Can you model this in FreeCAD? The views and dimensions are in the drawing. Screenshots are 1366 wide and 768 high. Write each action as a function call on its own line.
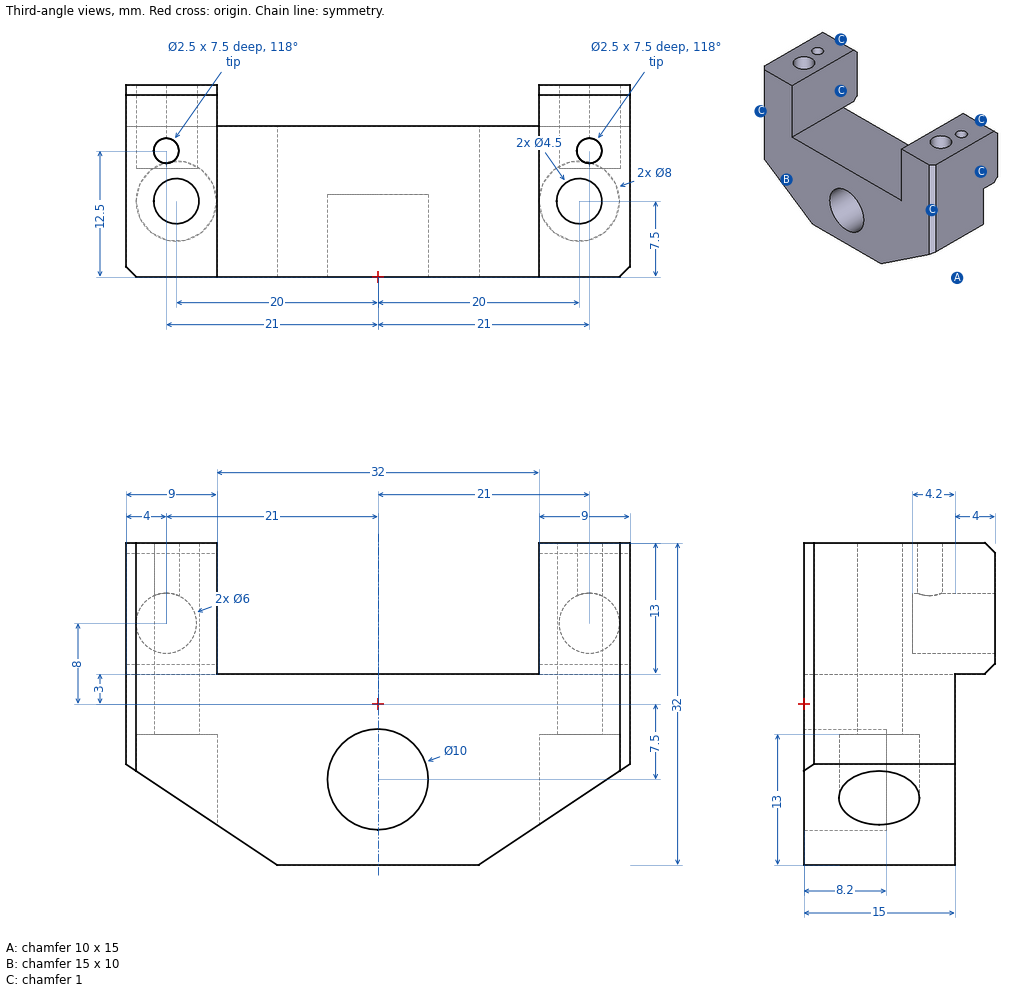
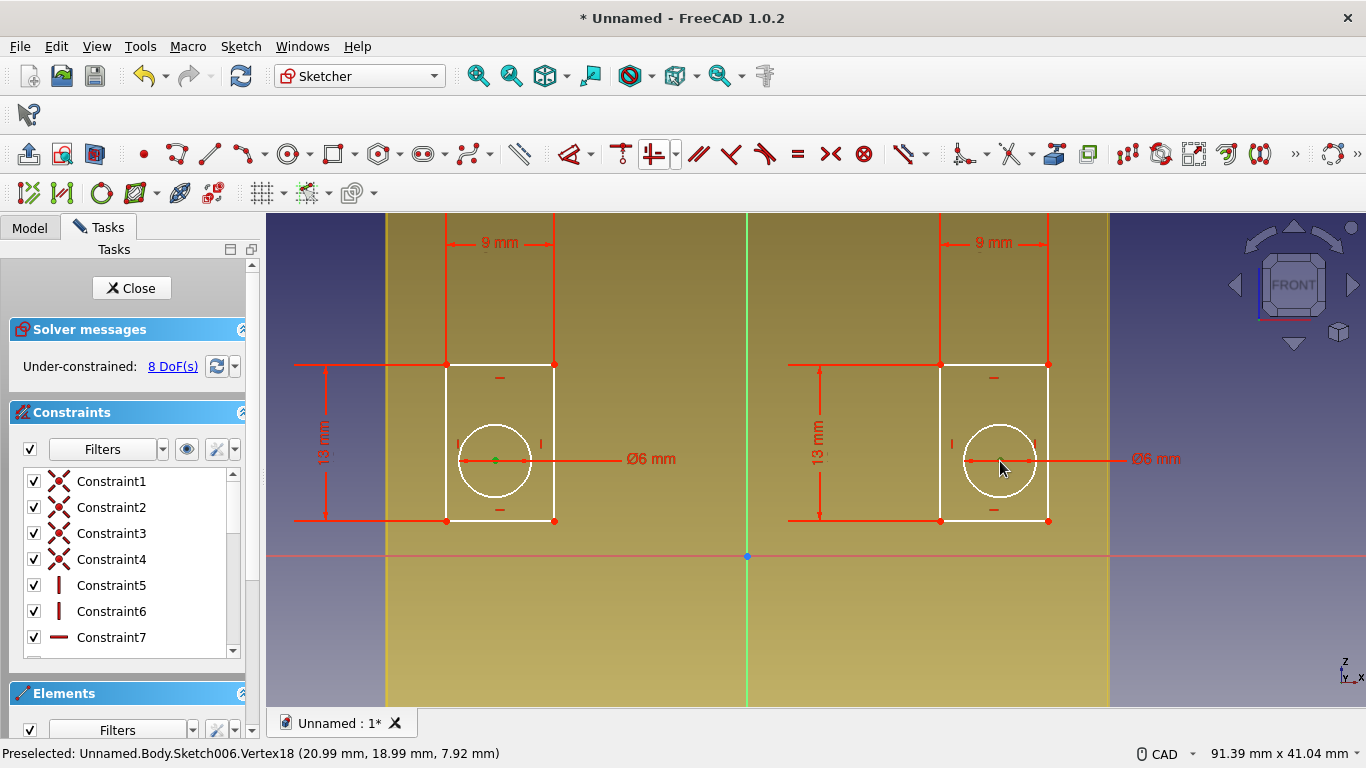
click(747, 648)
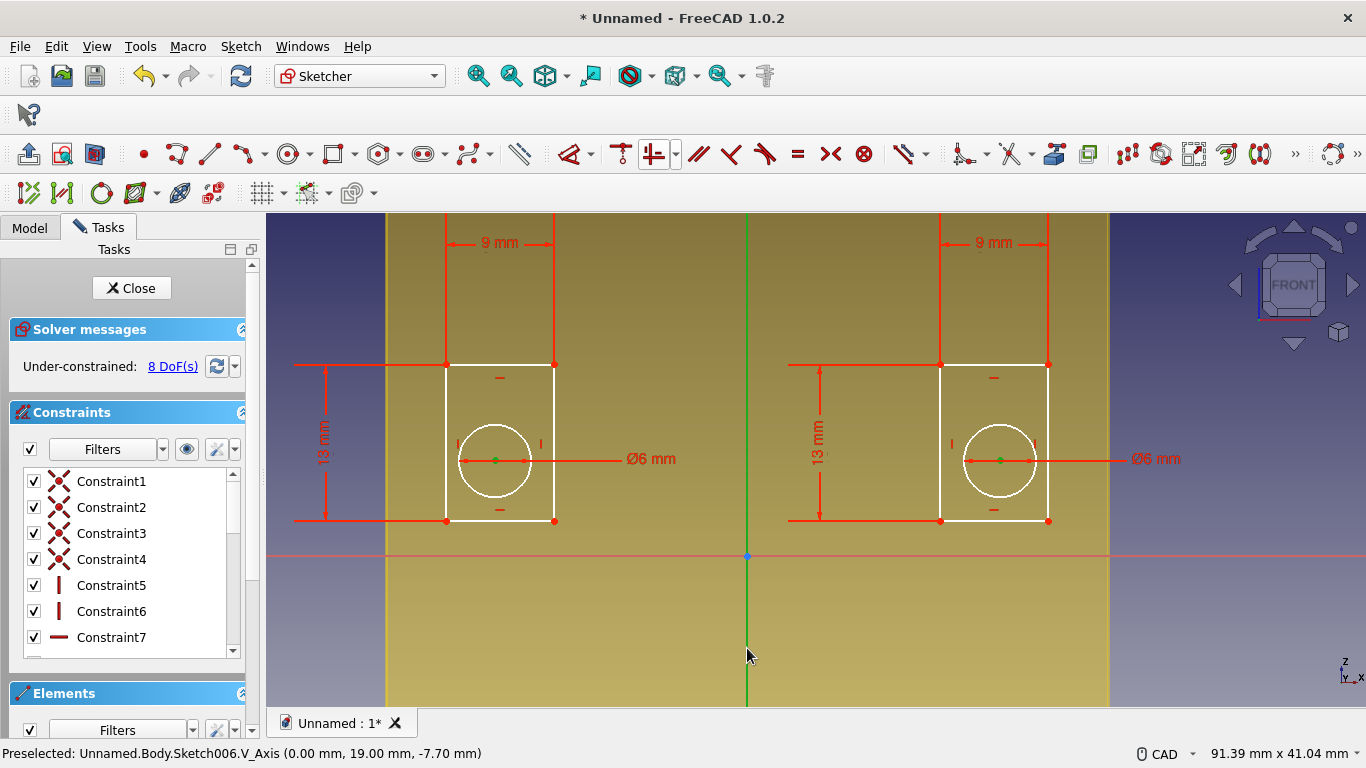
click(831, 154)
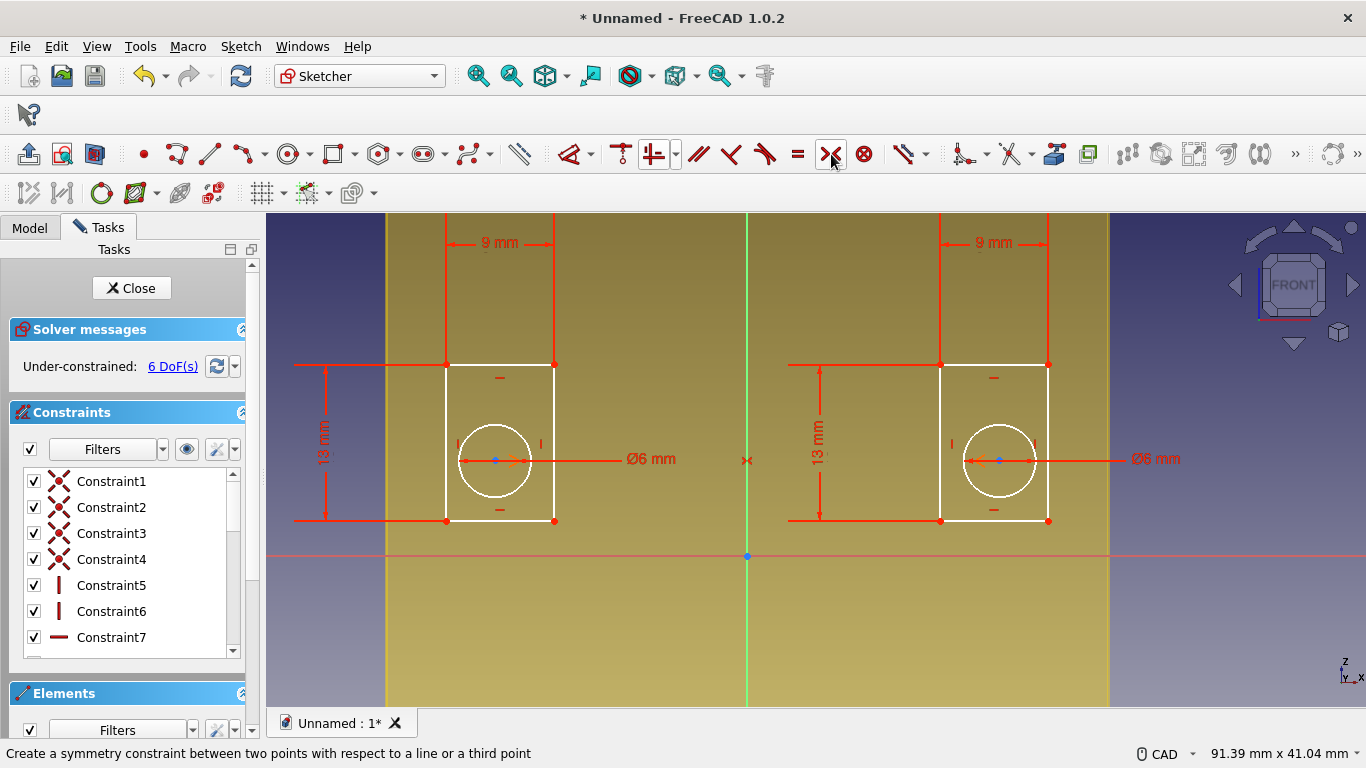
click(554, 365)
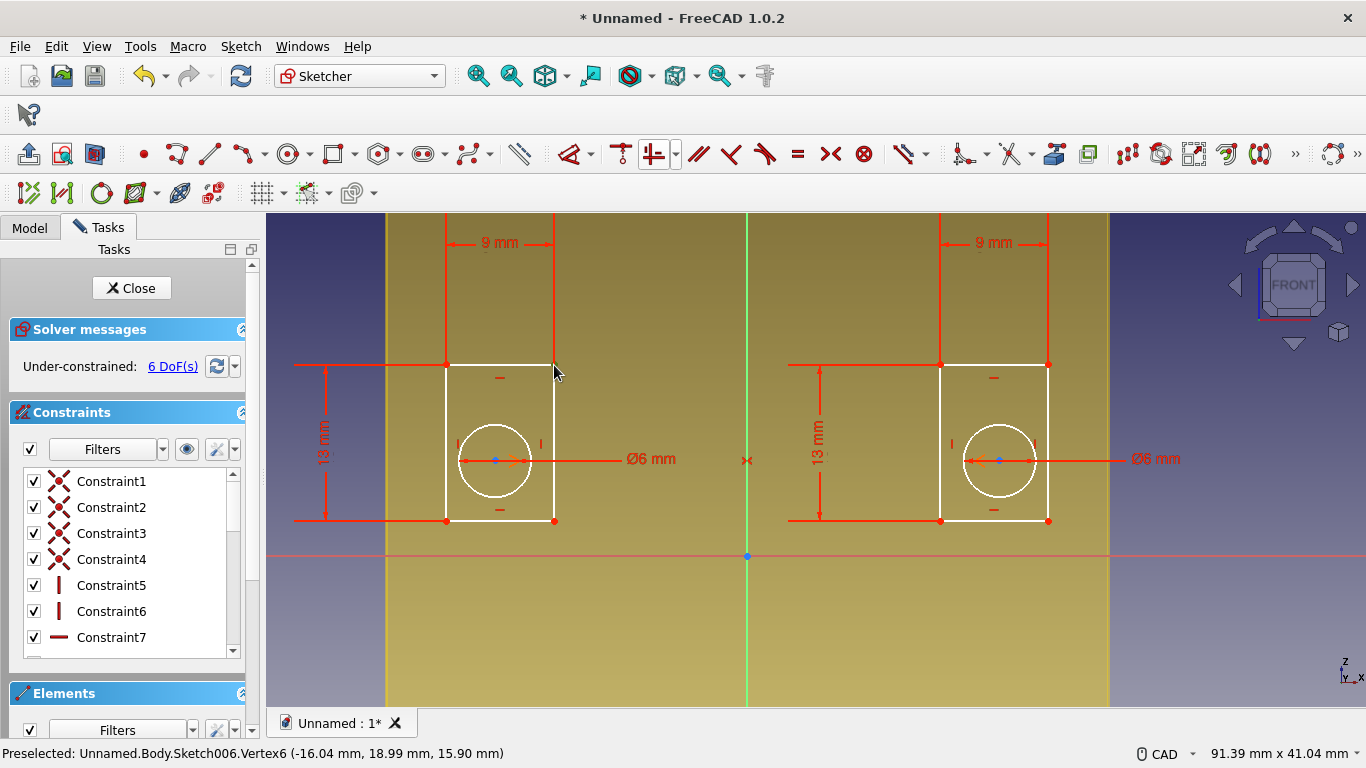
click(940, 365)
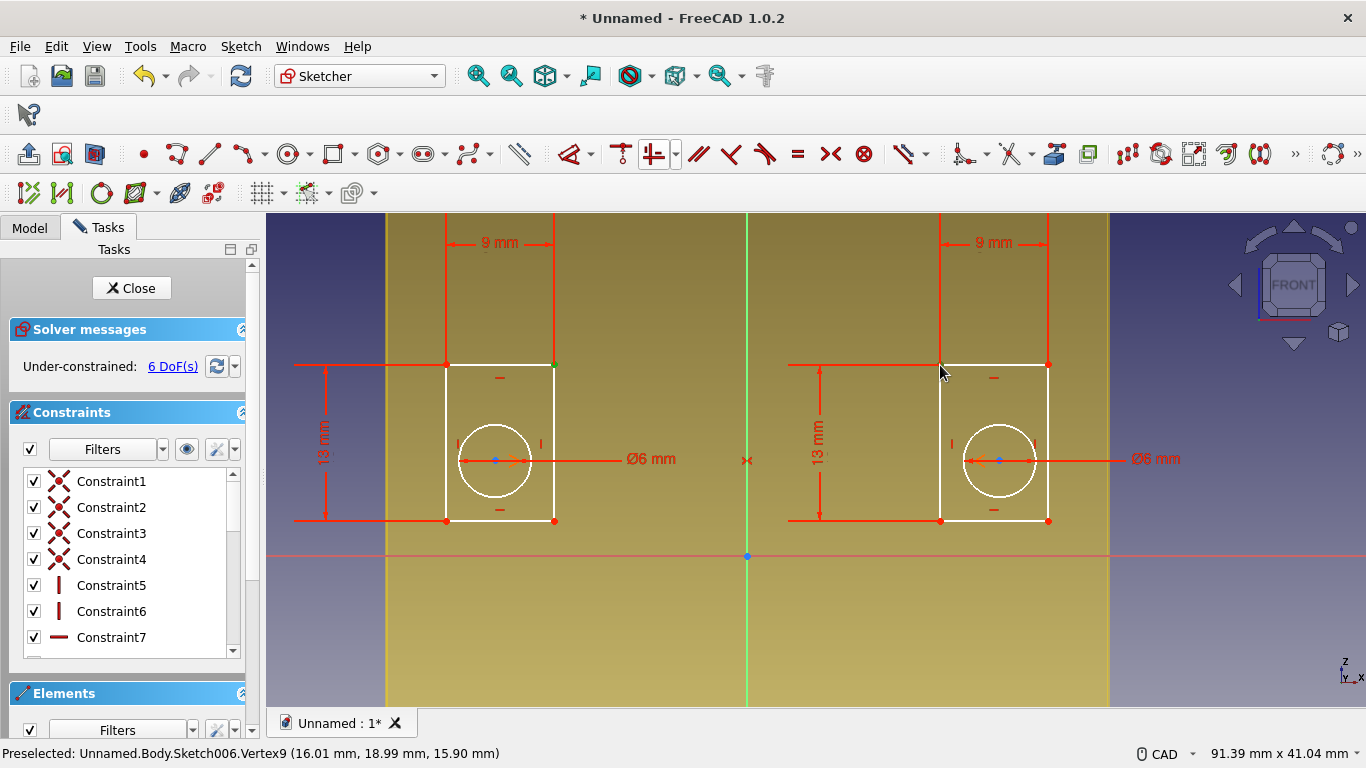
click(747, 648)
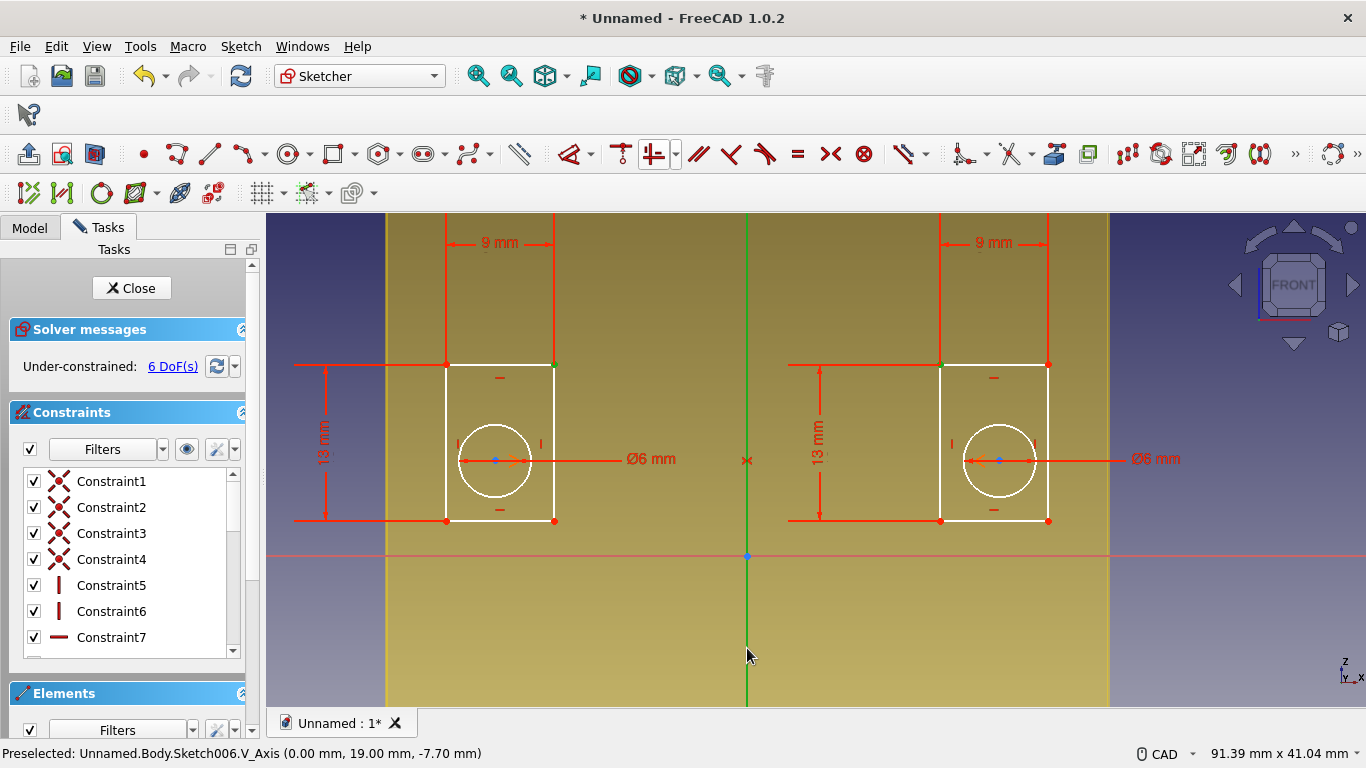
click(831, 154)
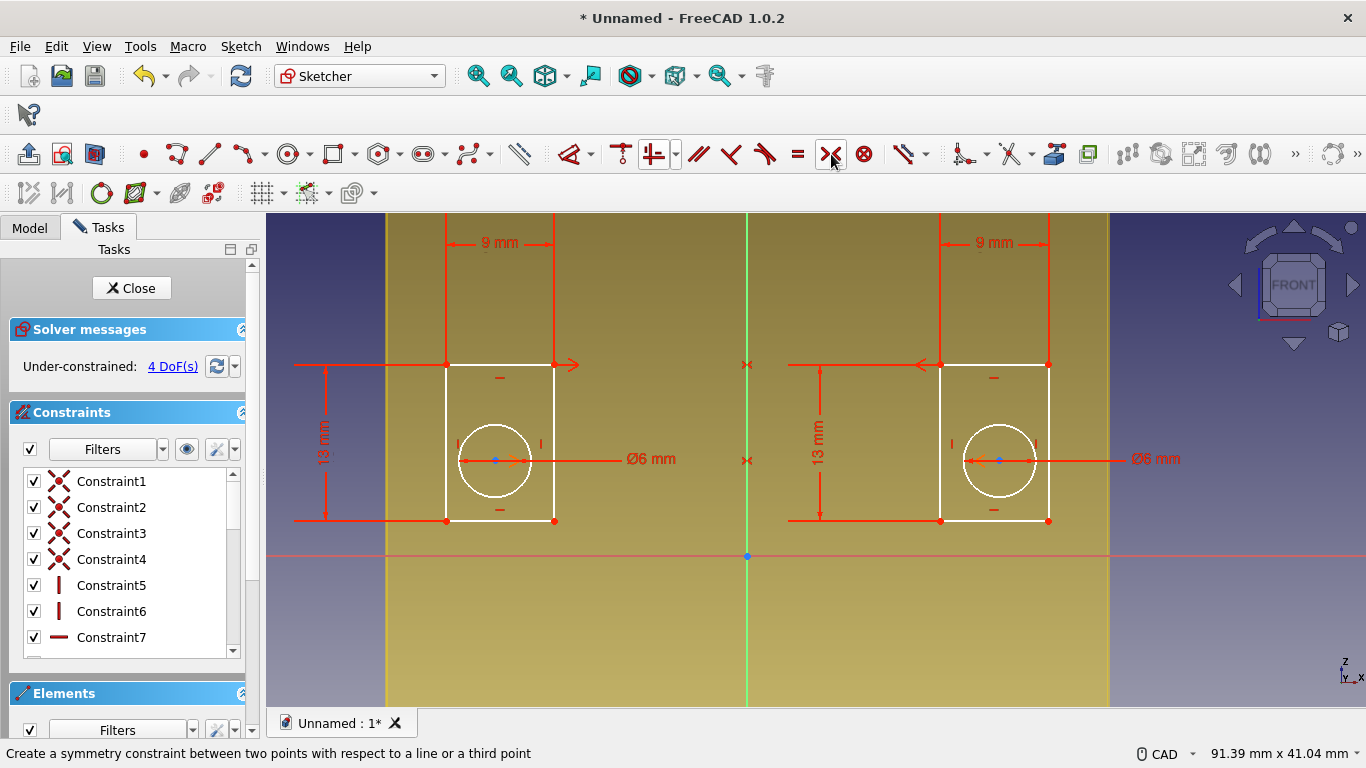
click(568, 154)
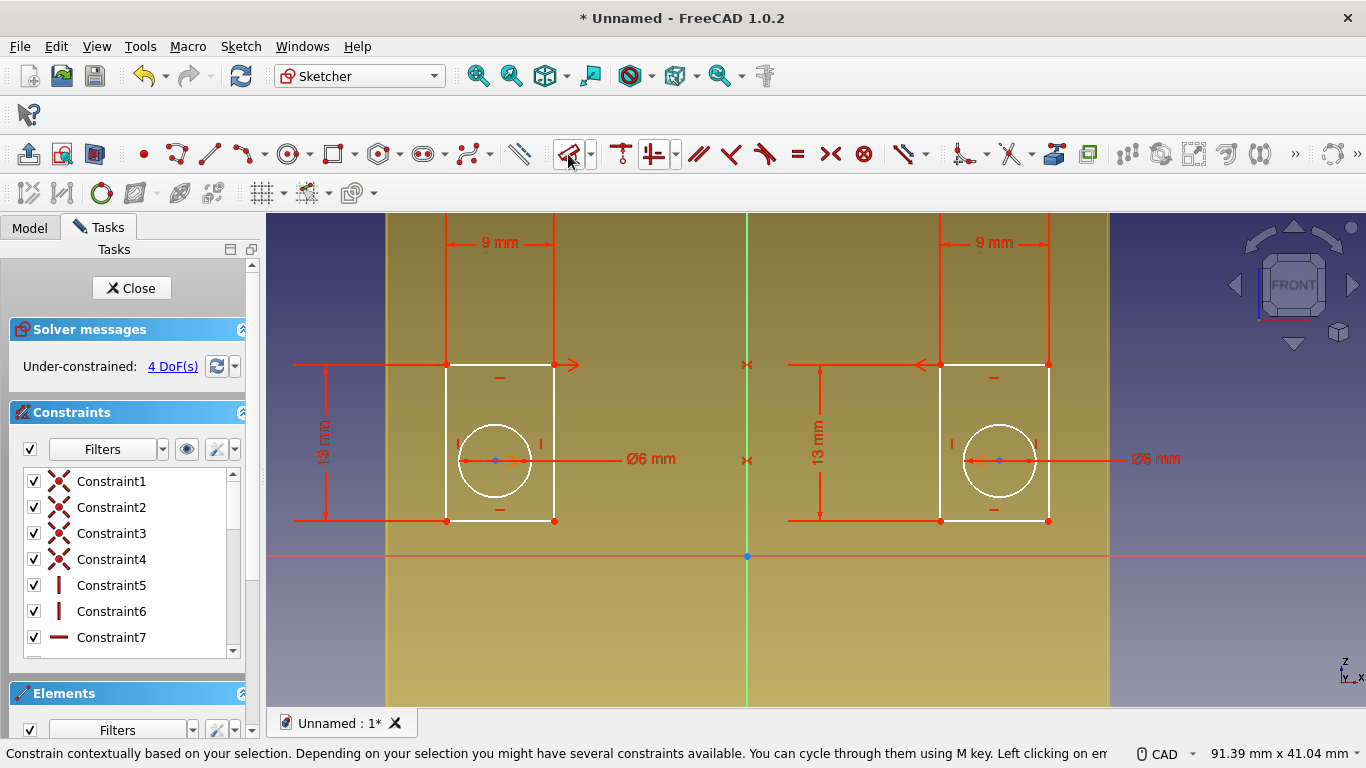
click(495, 461)
click(461, 542)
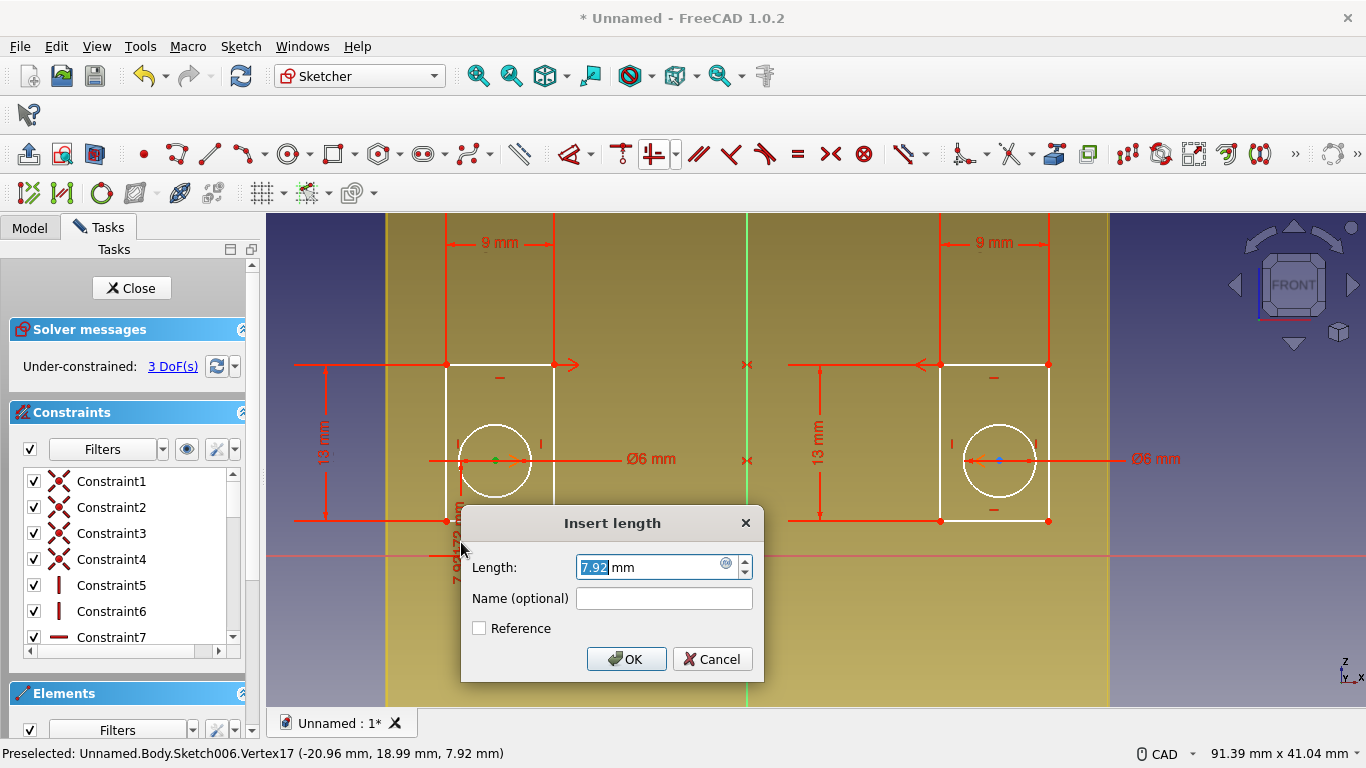
text(8)
key(Return)